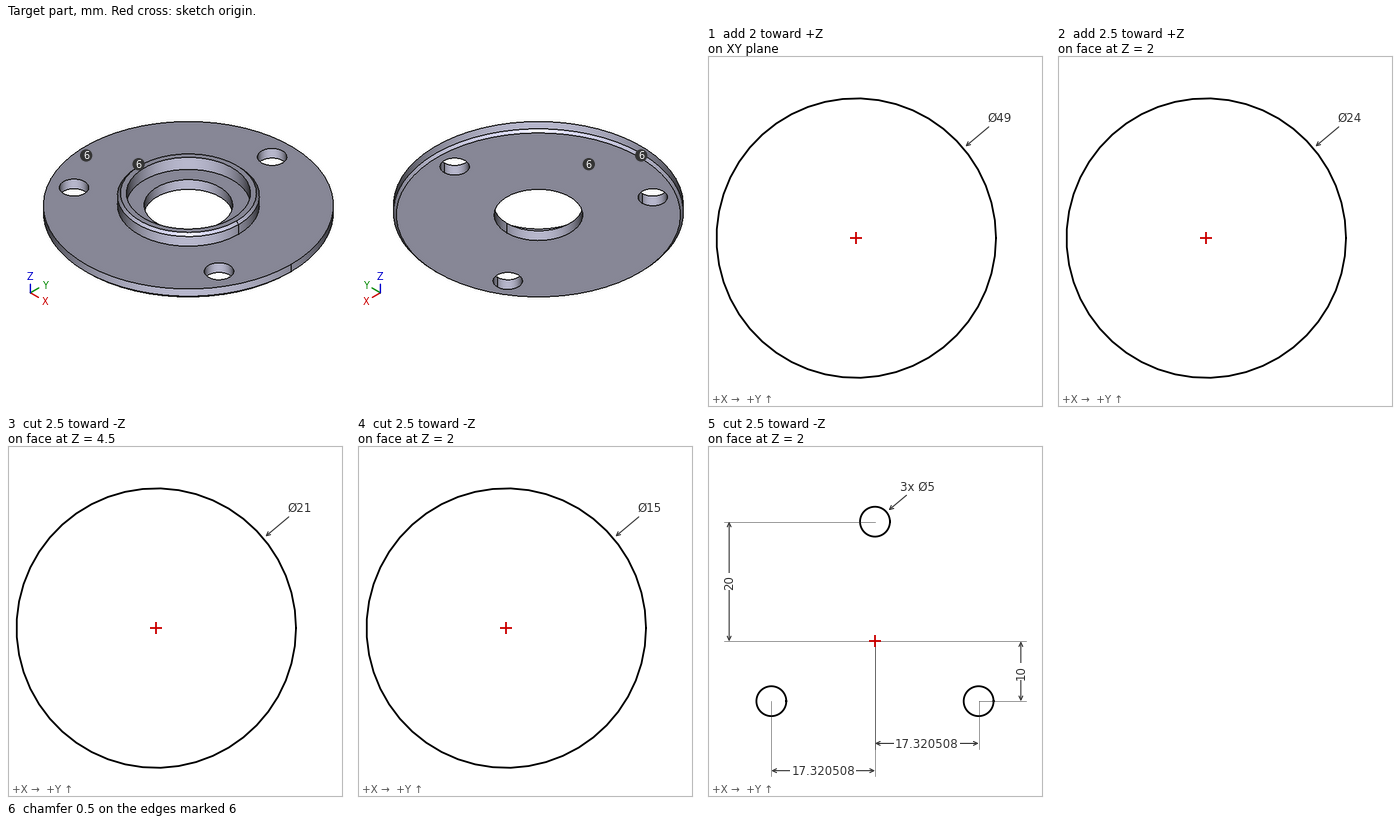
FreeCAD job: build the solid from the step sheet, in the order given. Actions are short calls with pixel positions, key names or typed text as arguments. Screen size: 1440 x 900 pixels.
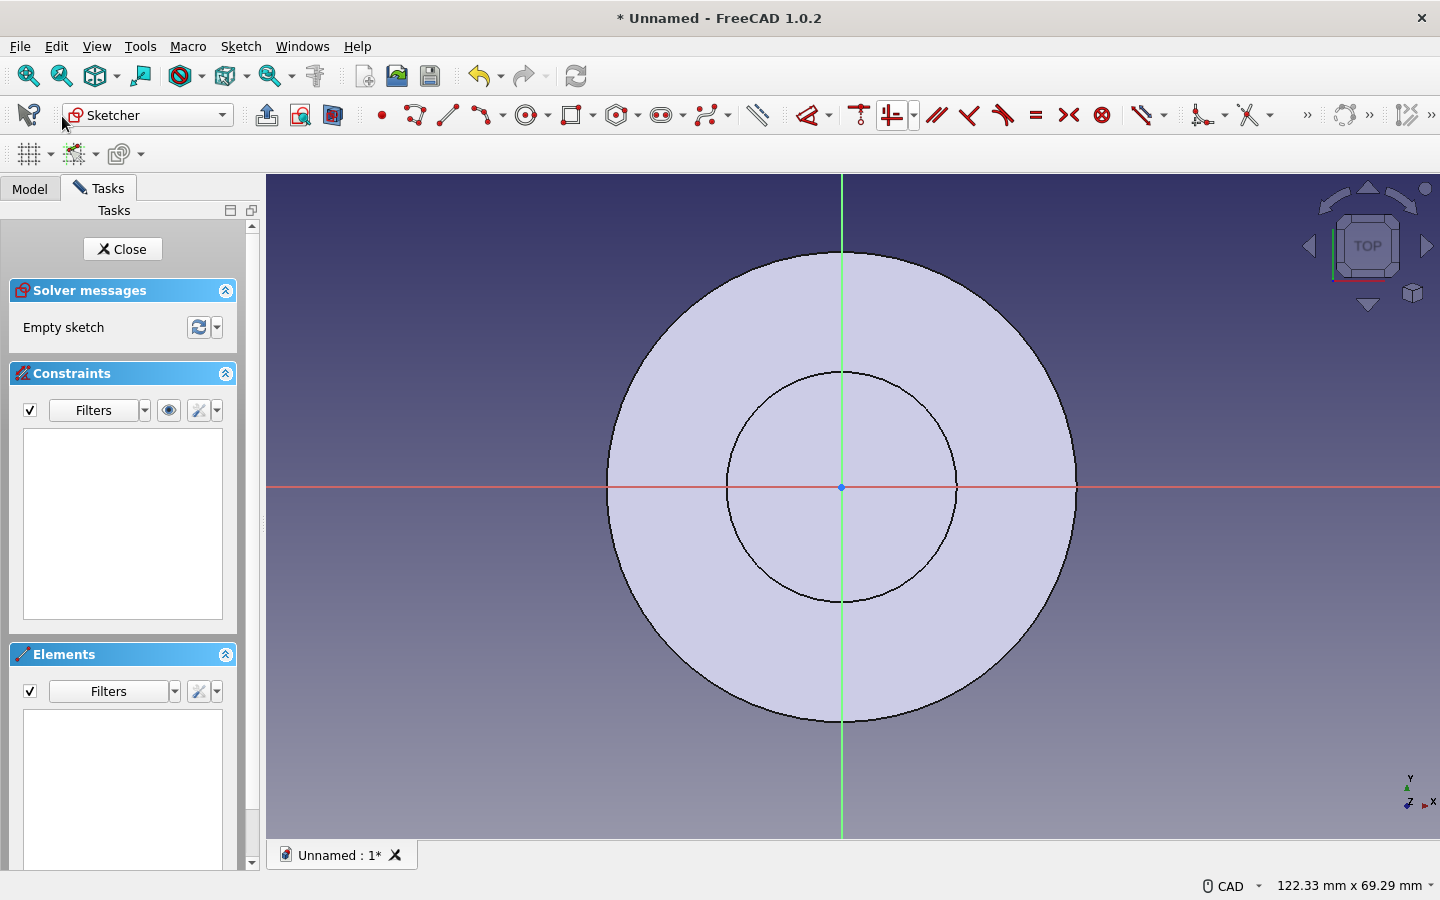
scroll(888, 471, up, 4)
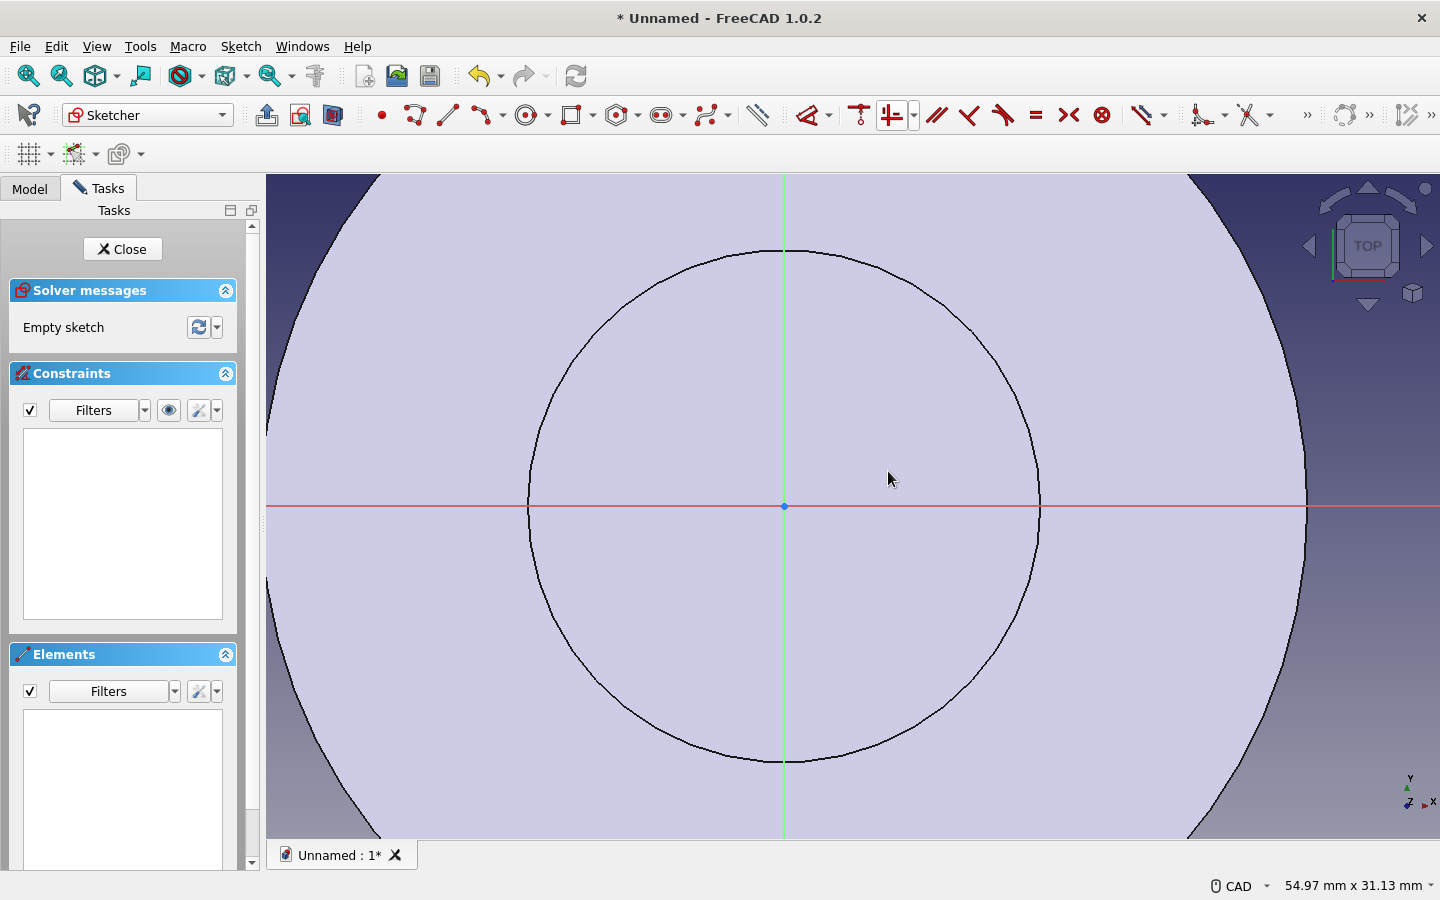
click(526, 116)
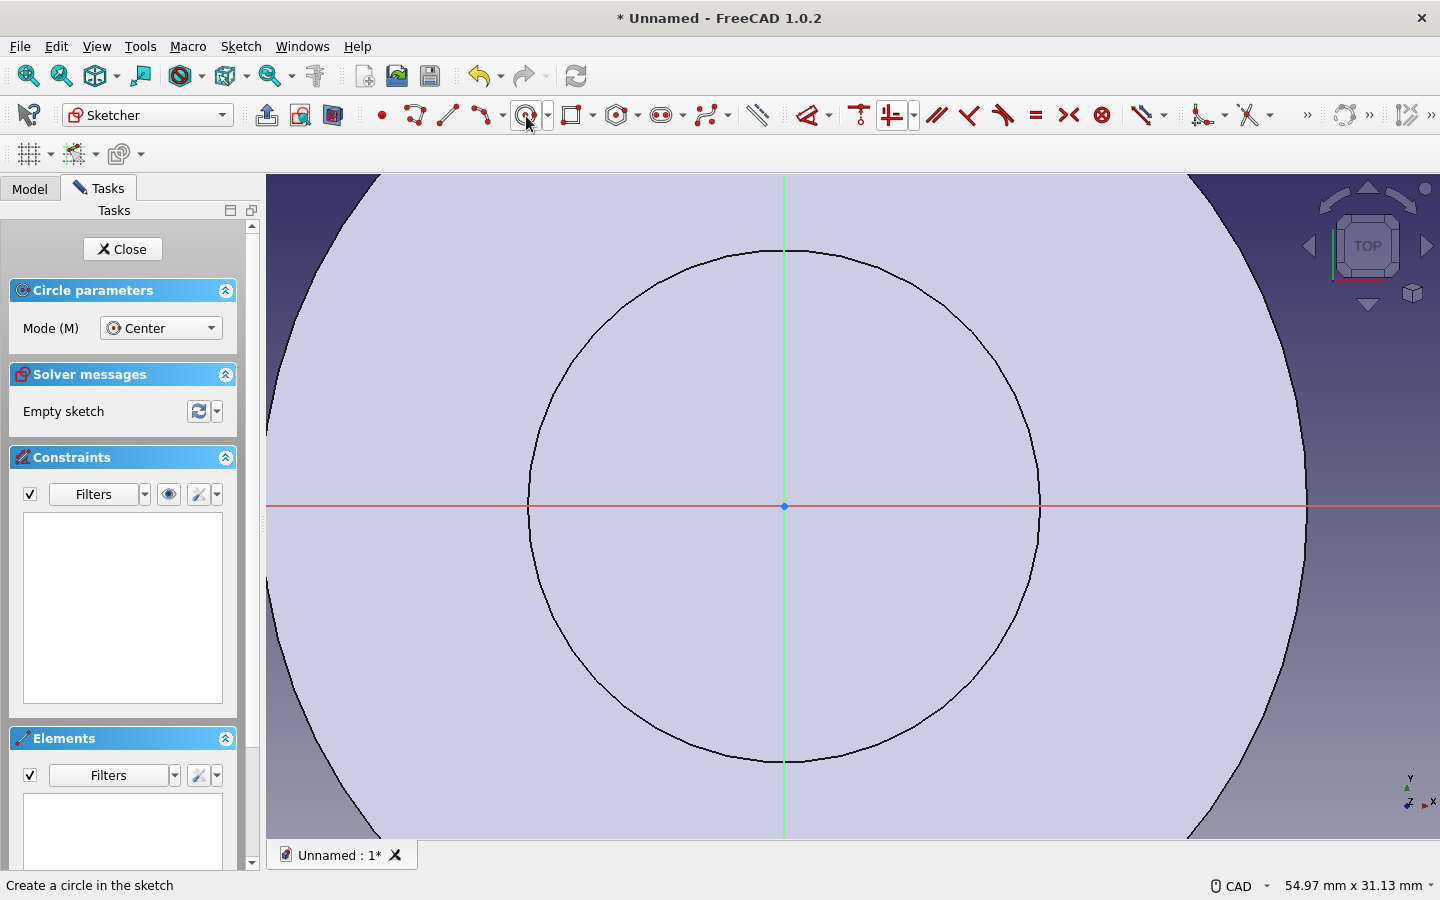
click(784, 506)
click(943, 348)
key(Escape)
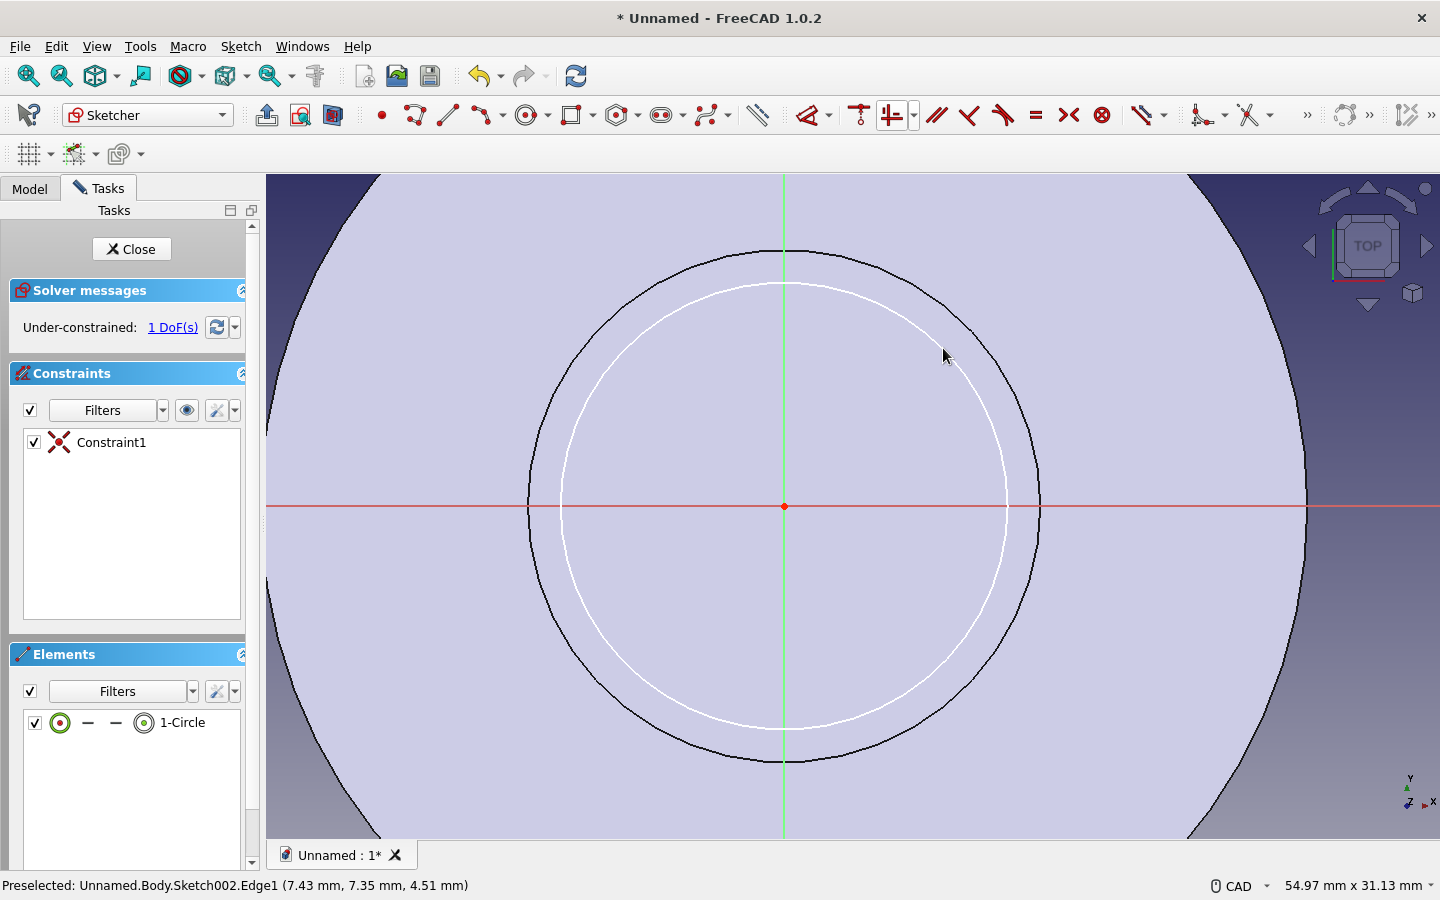
click(942, 348)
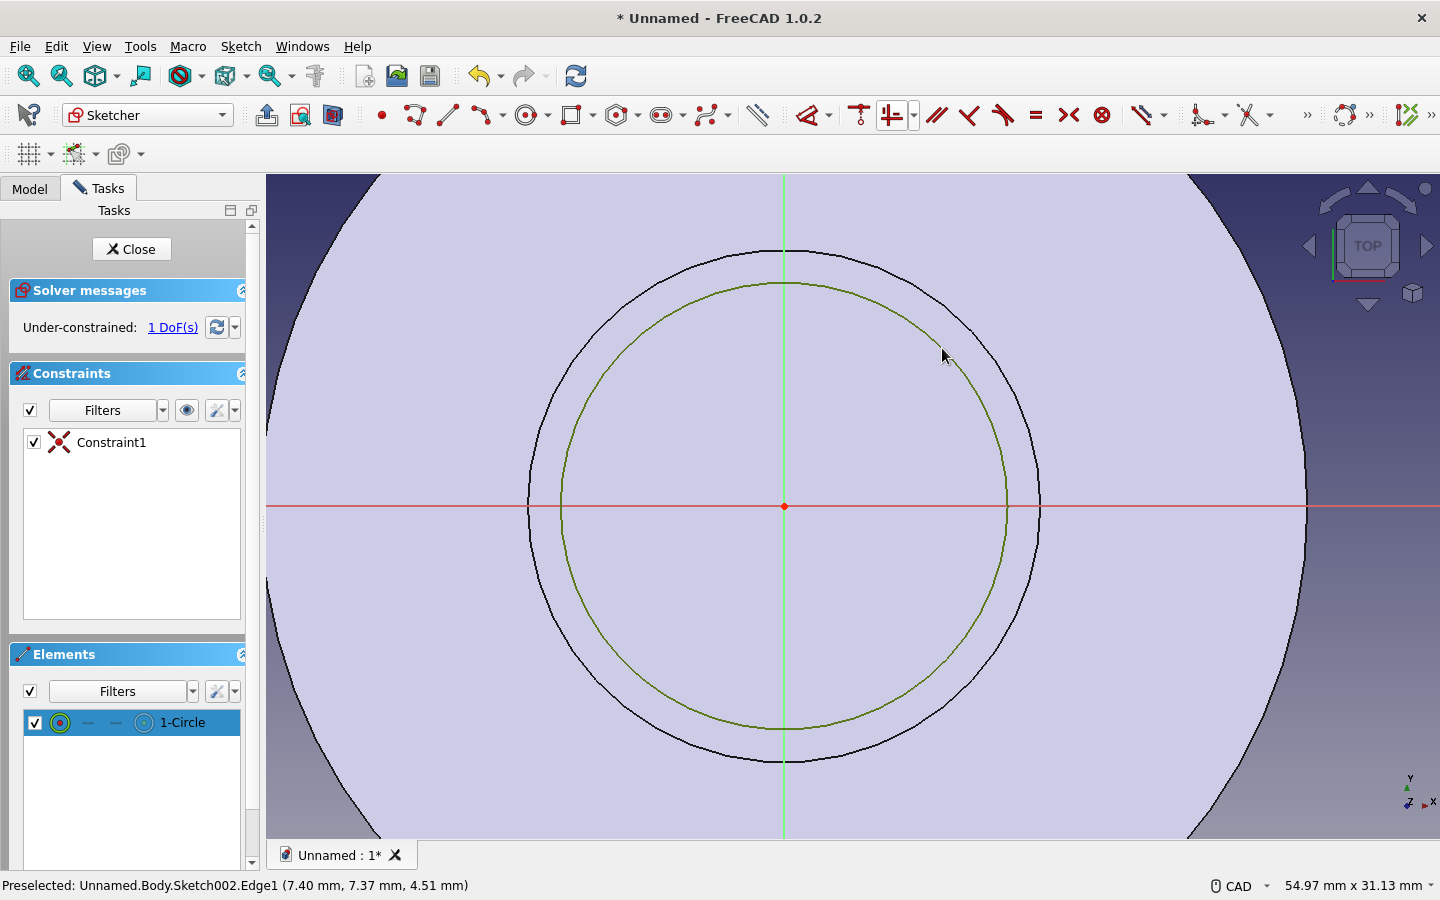
key(k)
key(o)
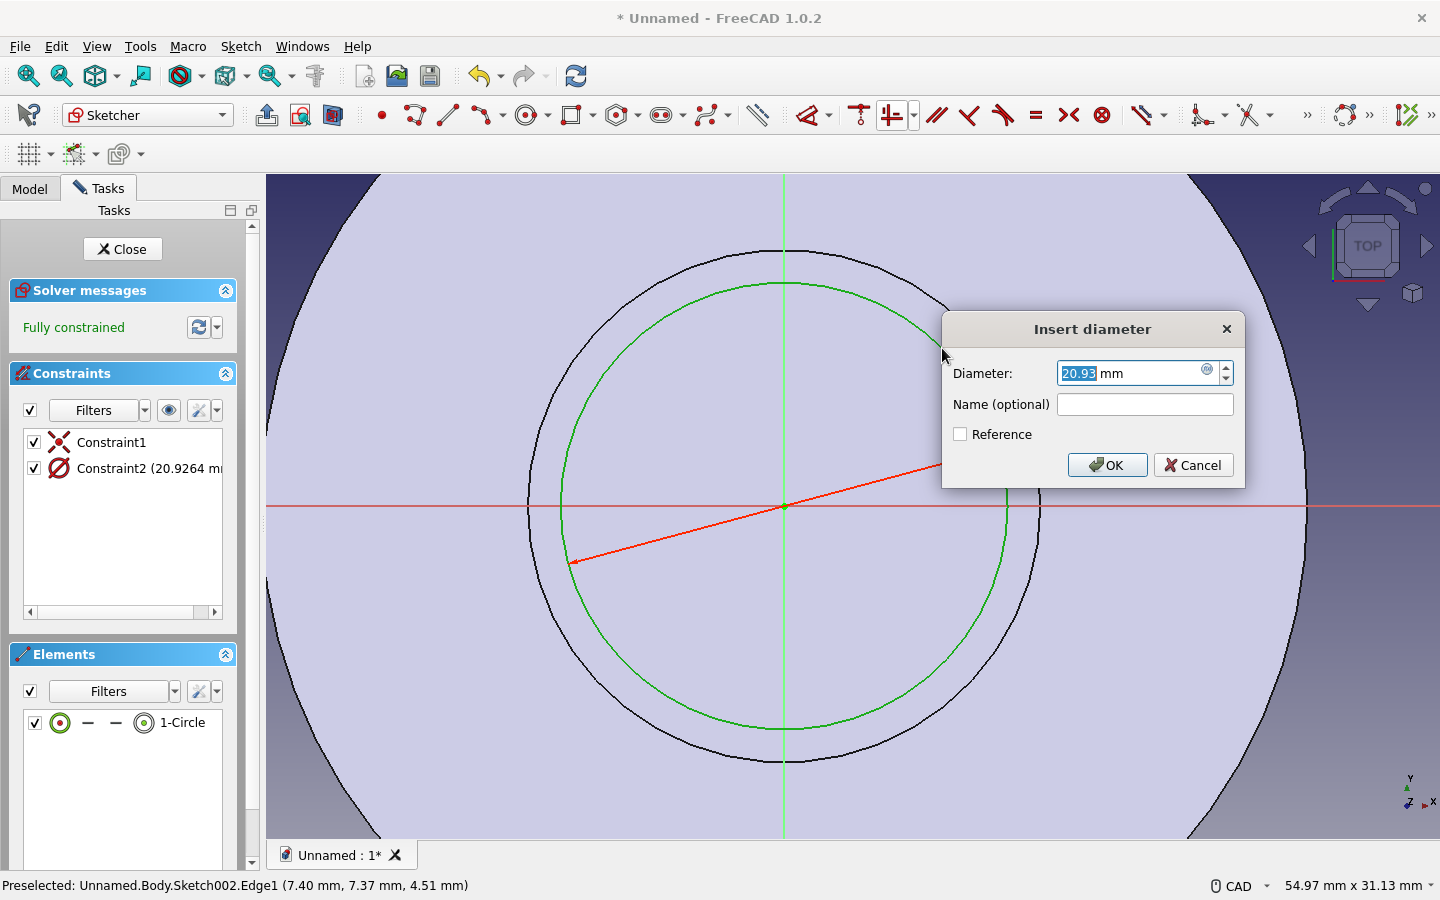
text(21)
key(Return)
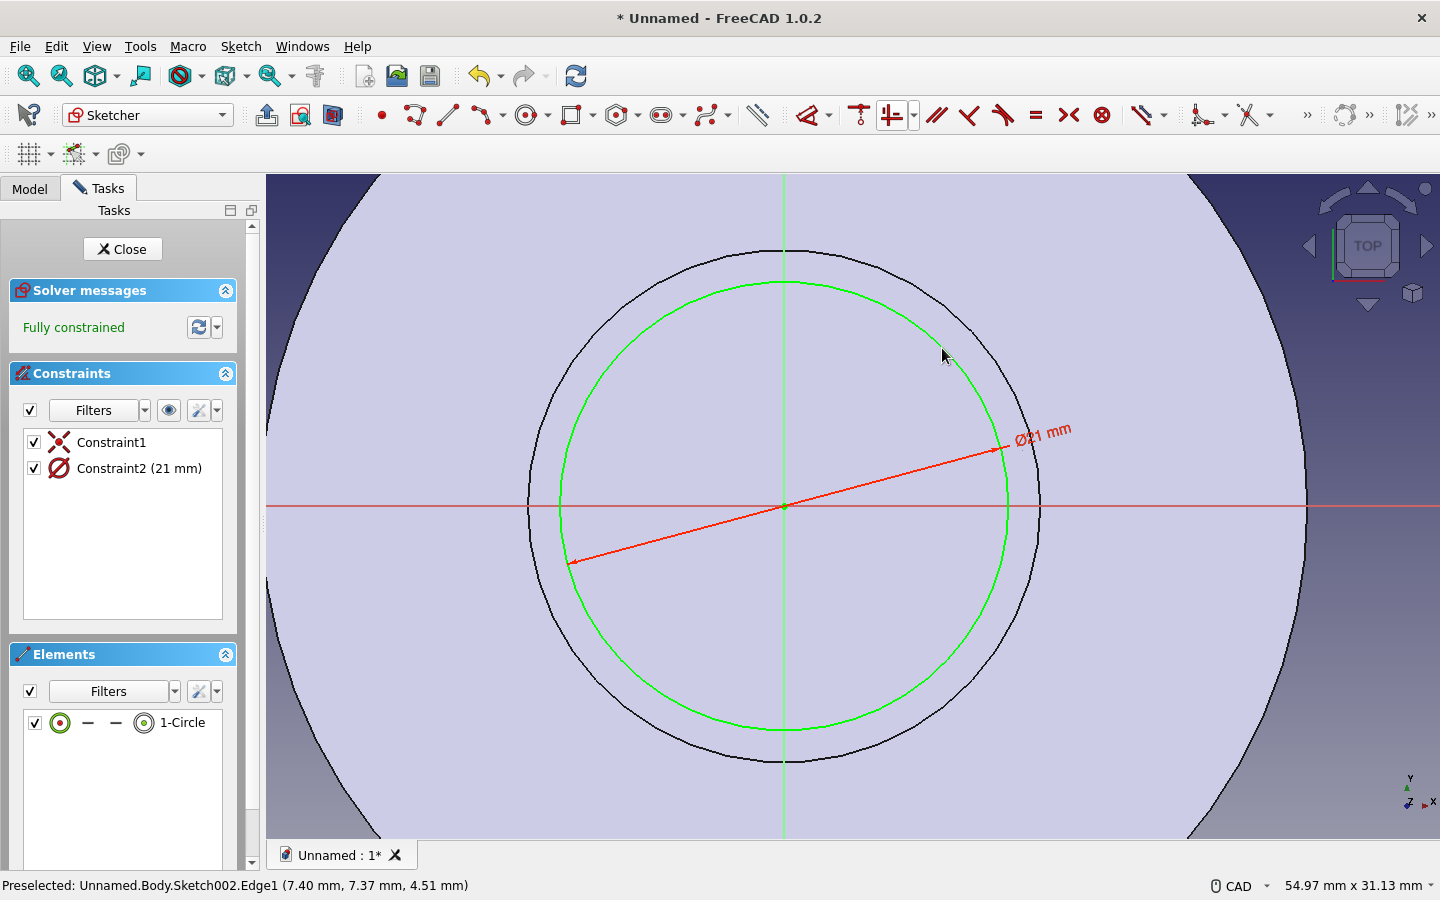
click(123, 249)